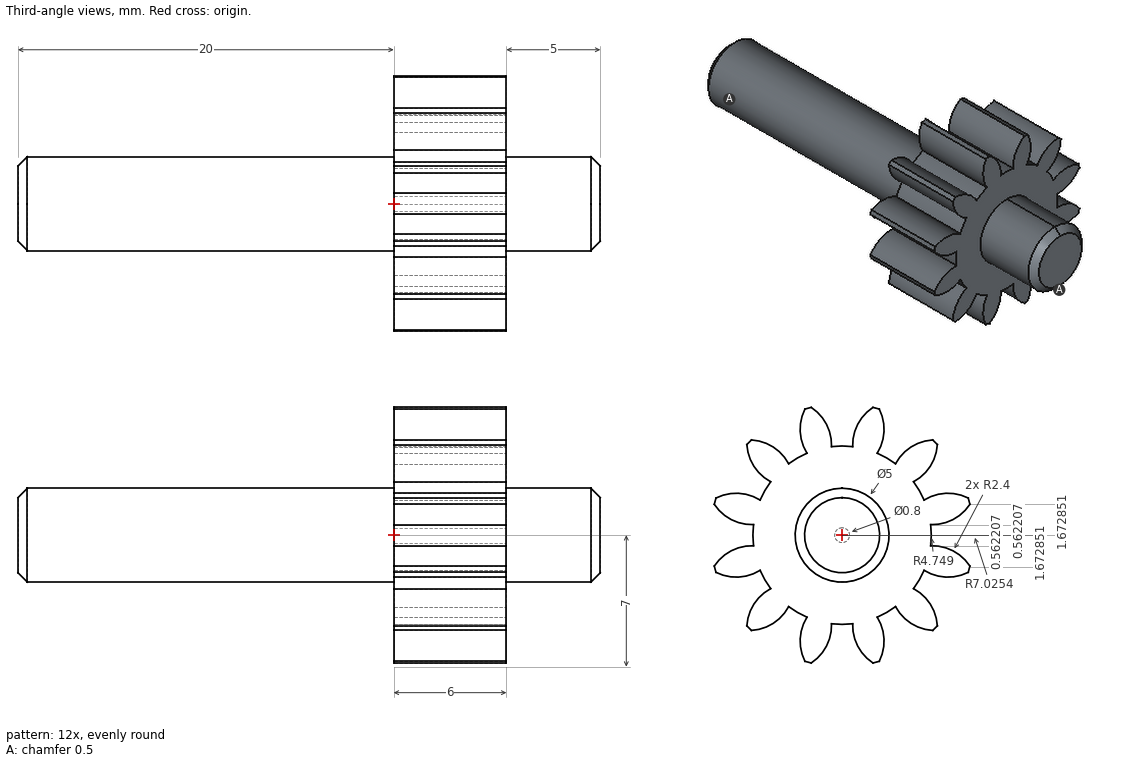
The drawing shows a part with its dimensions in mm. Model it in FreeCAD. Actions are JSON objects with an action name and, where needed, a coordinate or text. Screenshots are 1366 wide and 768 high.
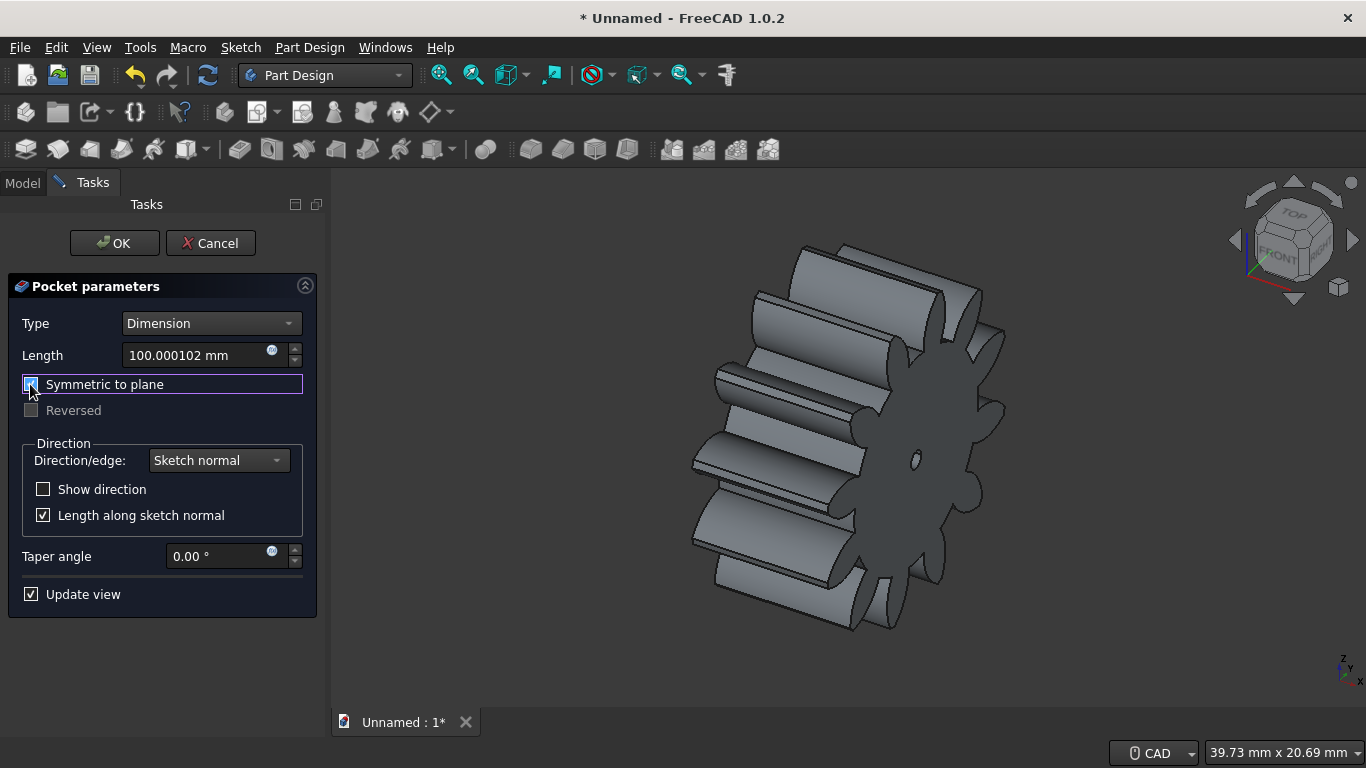
{"action": "left_click", "coordinate": [115, 243]}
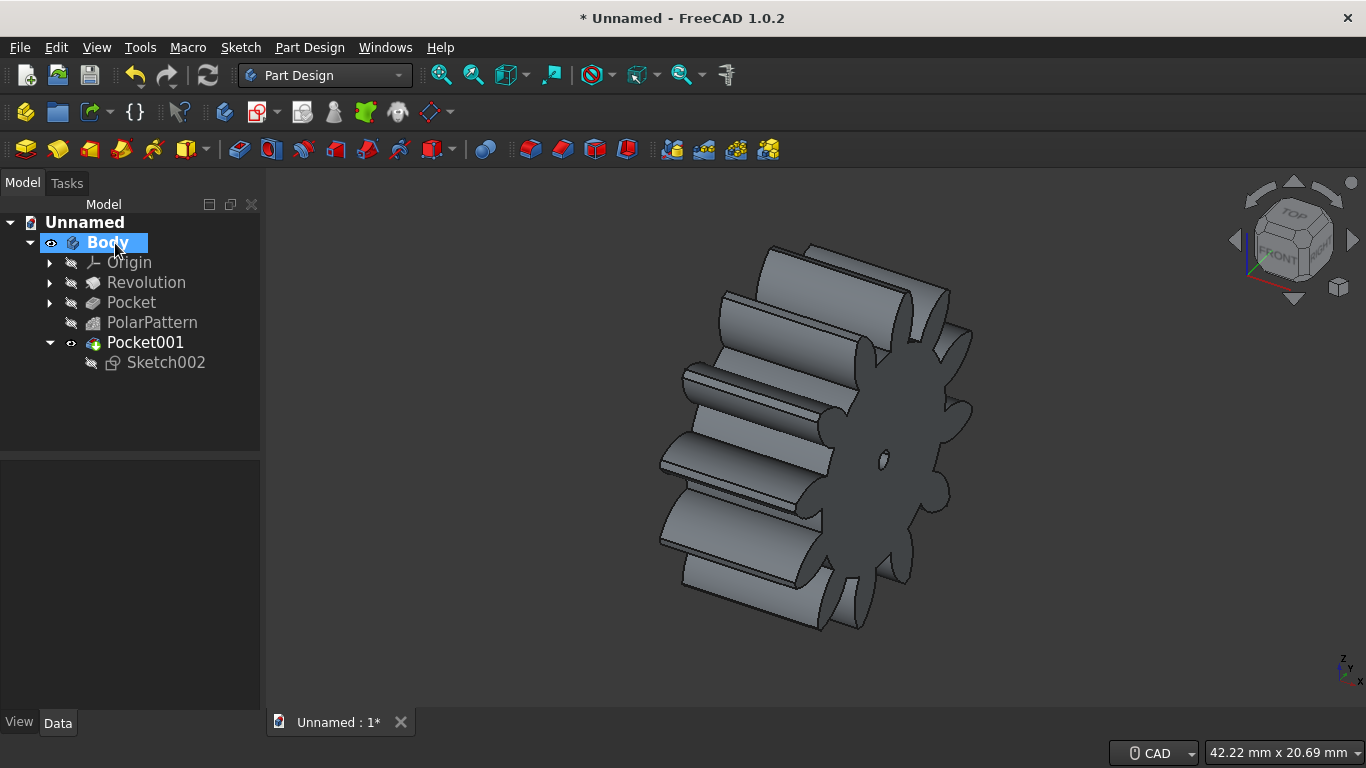
{"action": "left_click", "coordinate": [858, 443]}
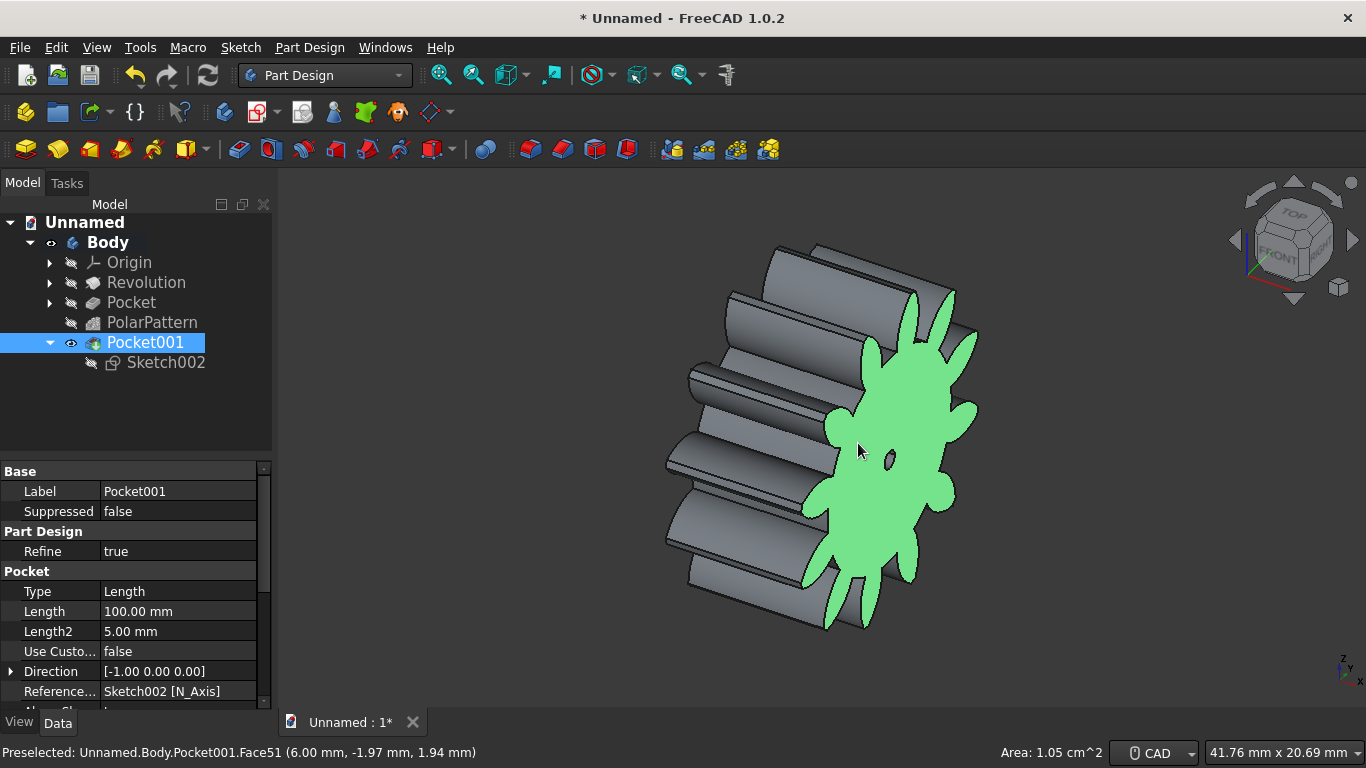
{"action": "left_click", "coordinate": [258, 112]}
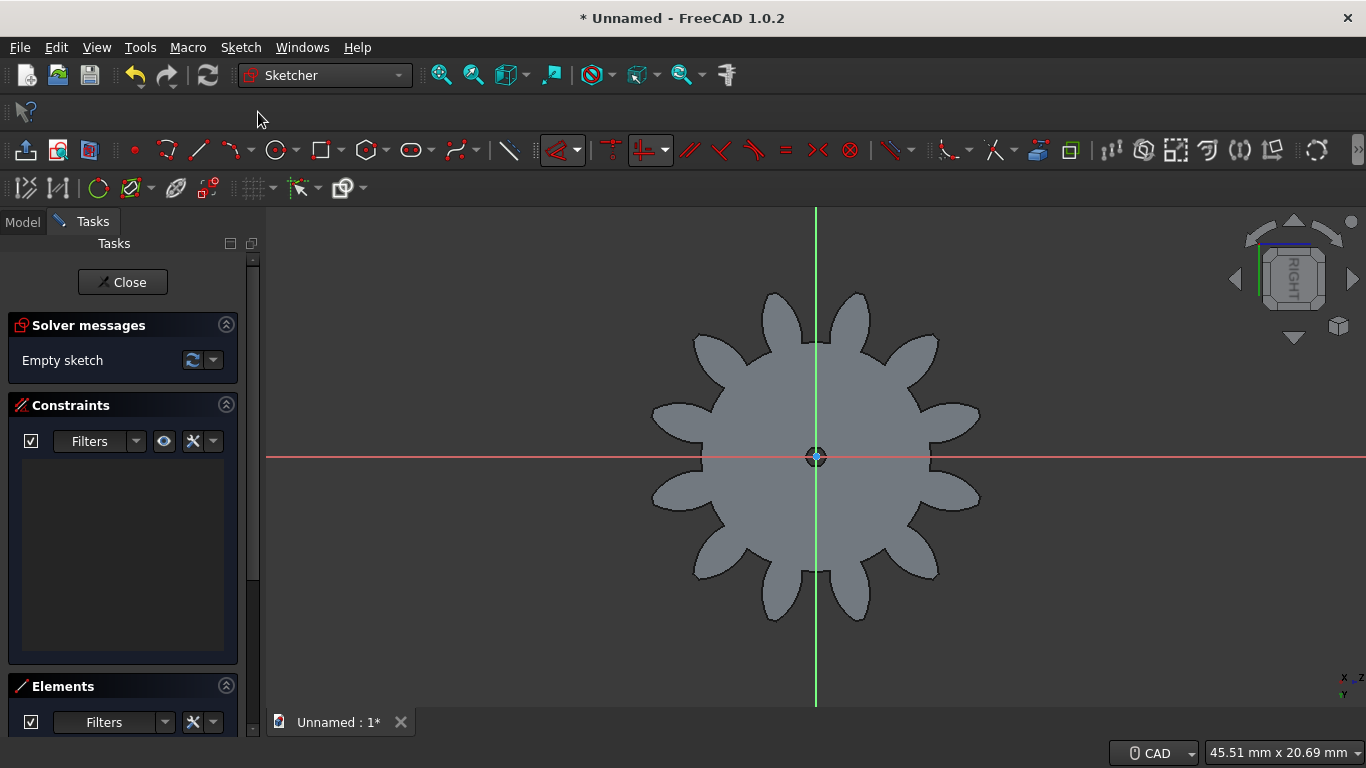
{"action": "scroll", "coordinate": [856, 457], "scroll_direction": "up", "scroll_amount": 5}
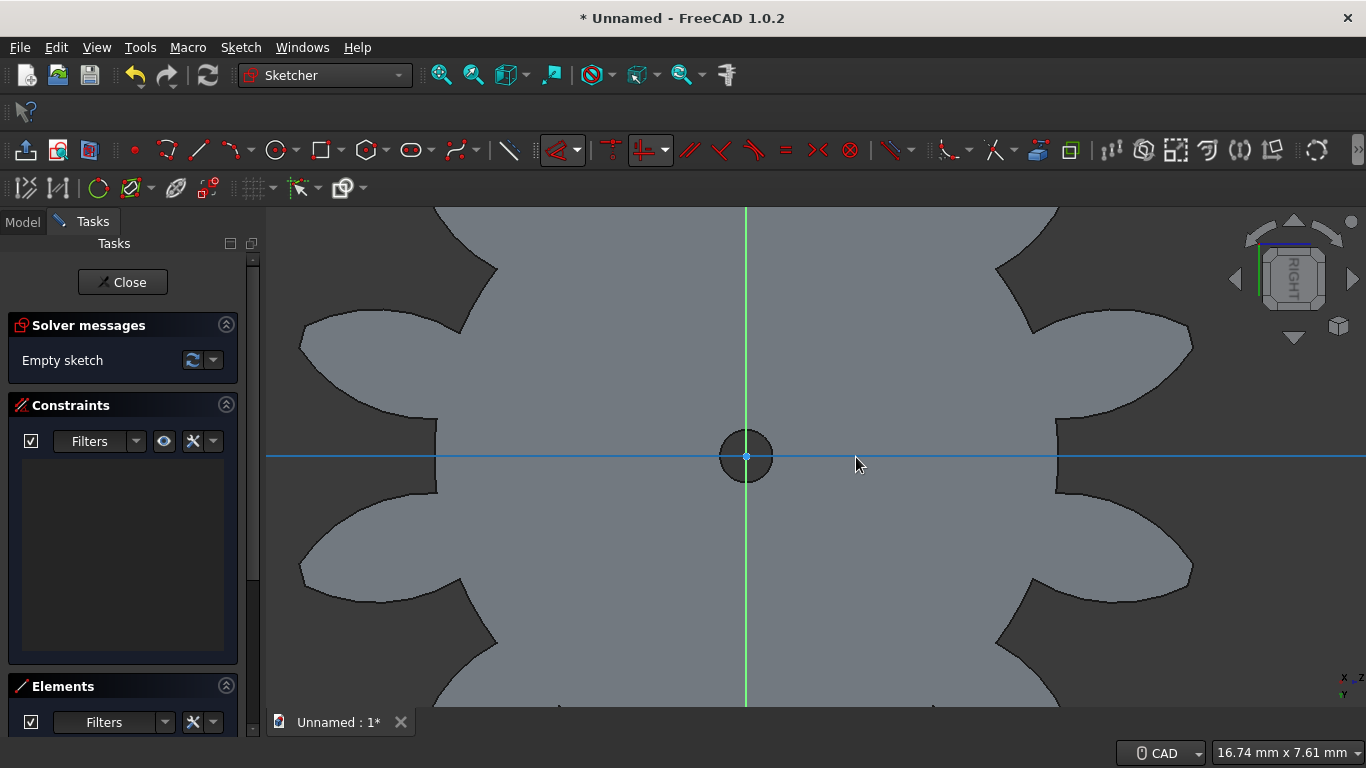
{"action": "left_click", "coordinate": [276, 150]}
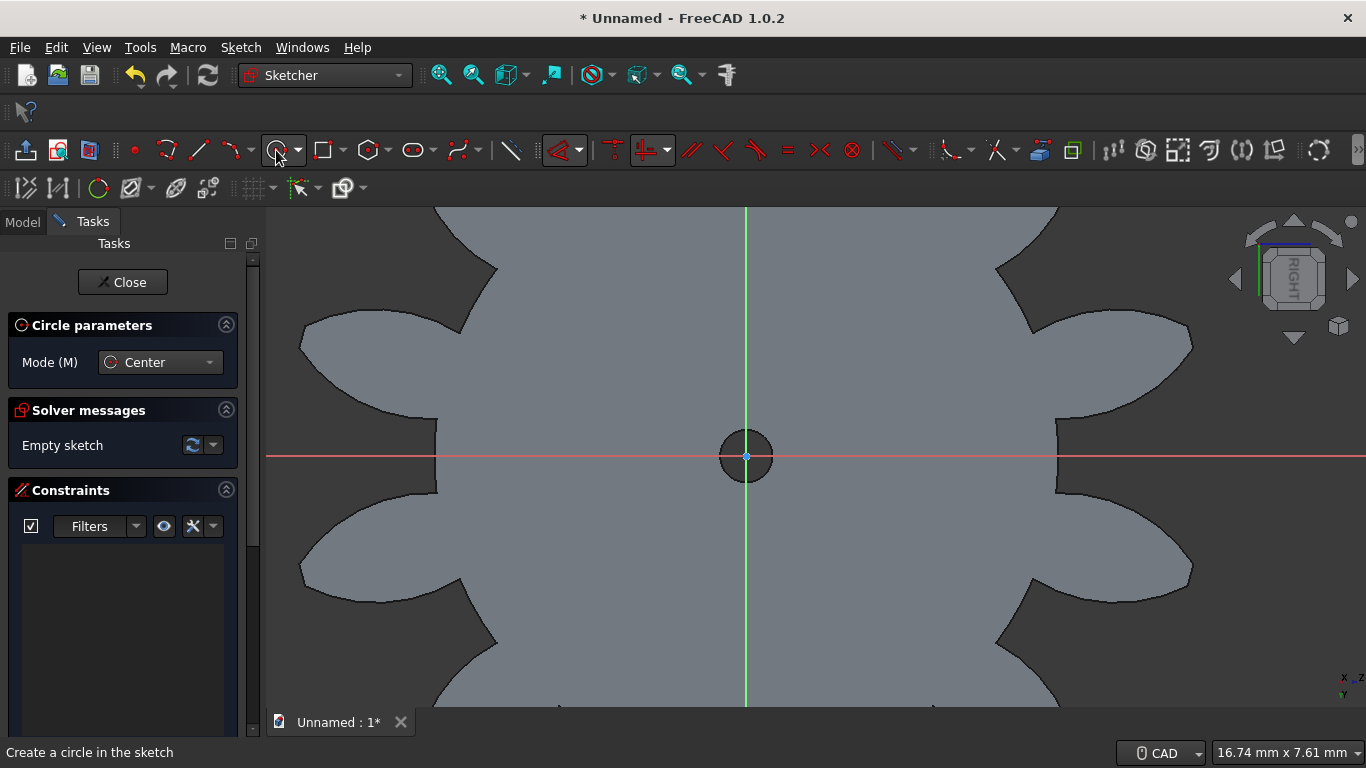
{"action": "left_click", "coordinate": [746, 456]}
{"action": "left_click", "coordinate": [862, 340]}
{"action": "key", "text": "Escape"}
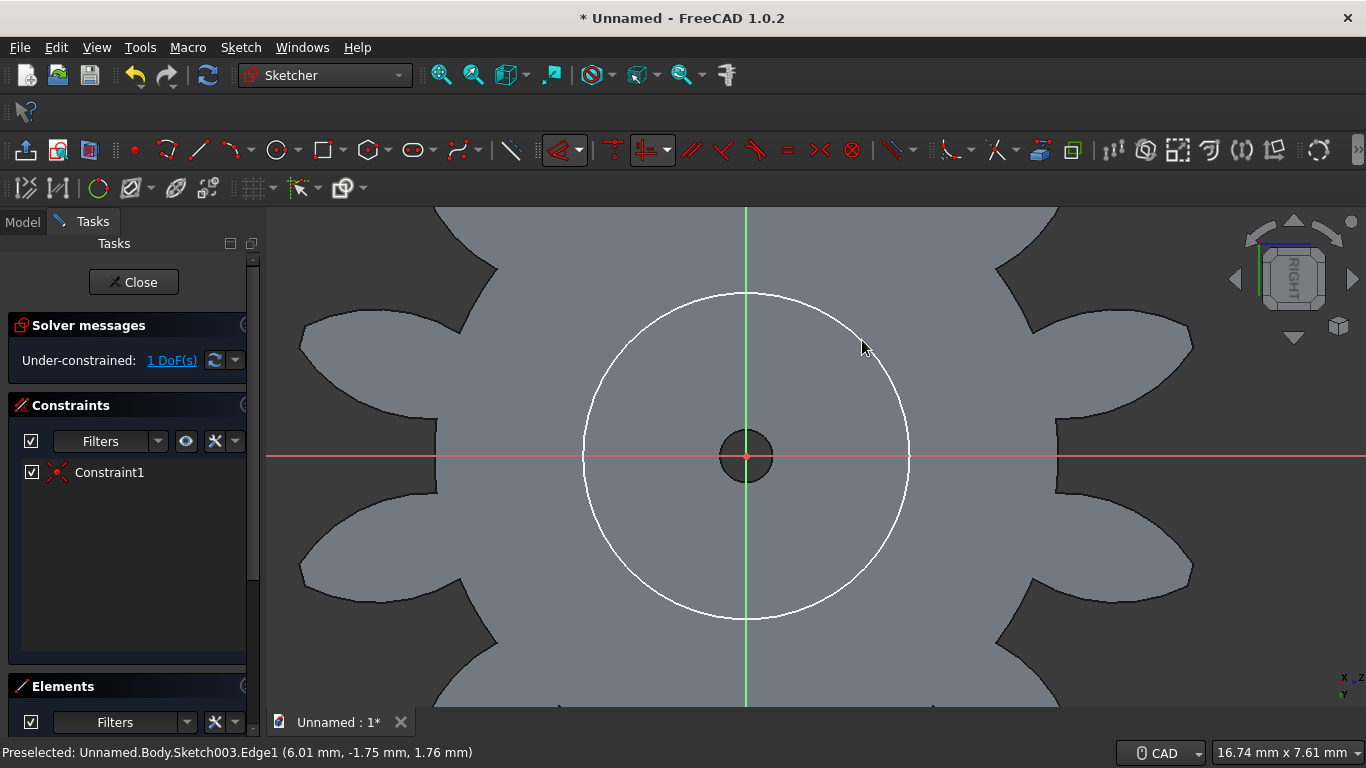
{"action": "left_click", "coordinate": [861, 340]}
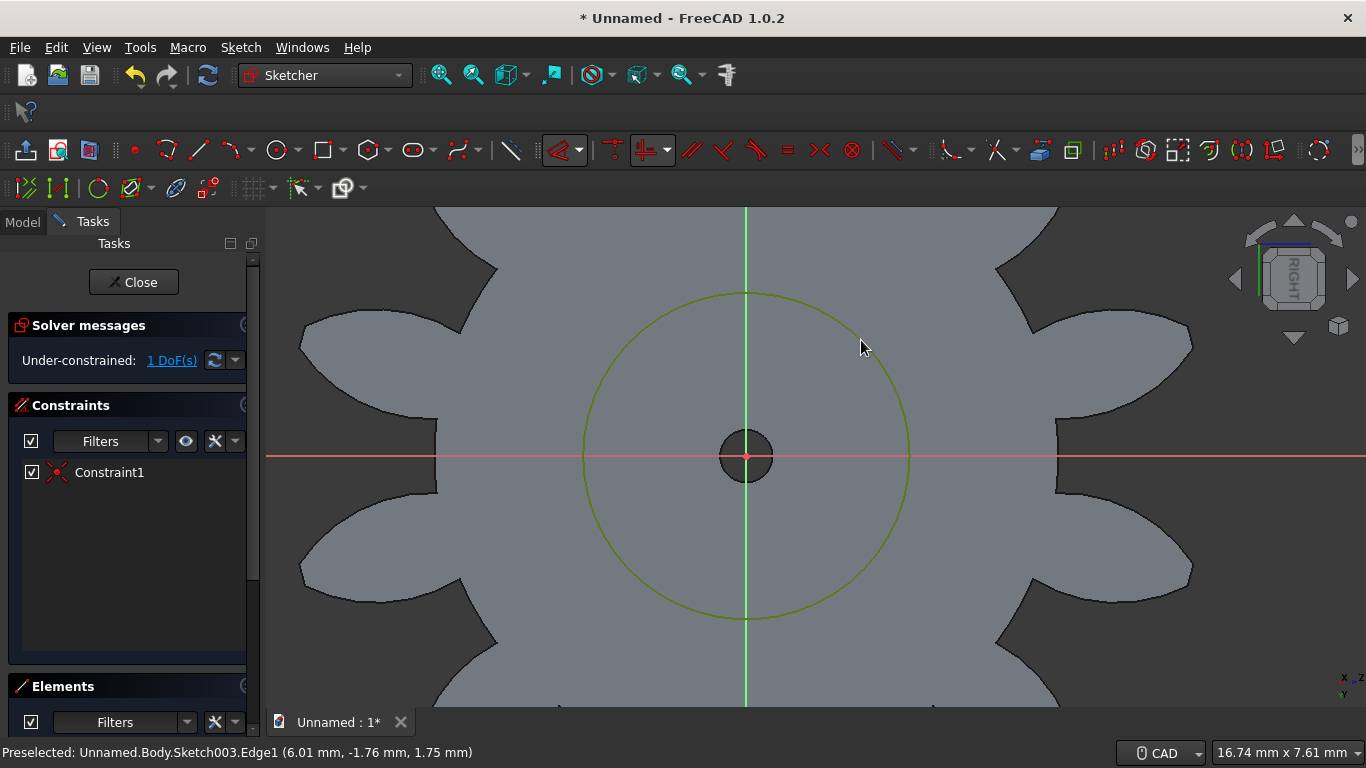
{"action": "left_click", "coordinate": [582, 150]}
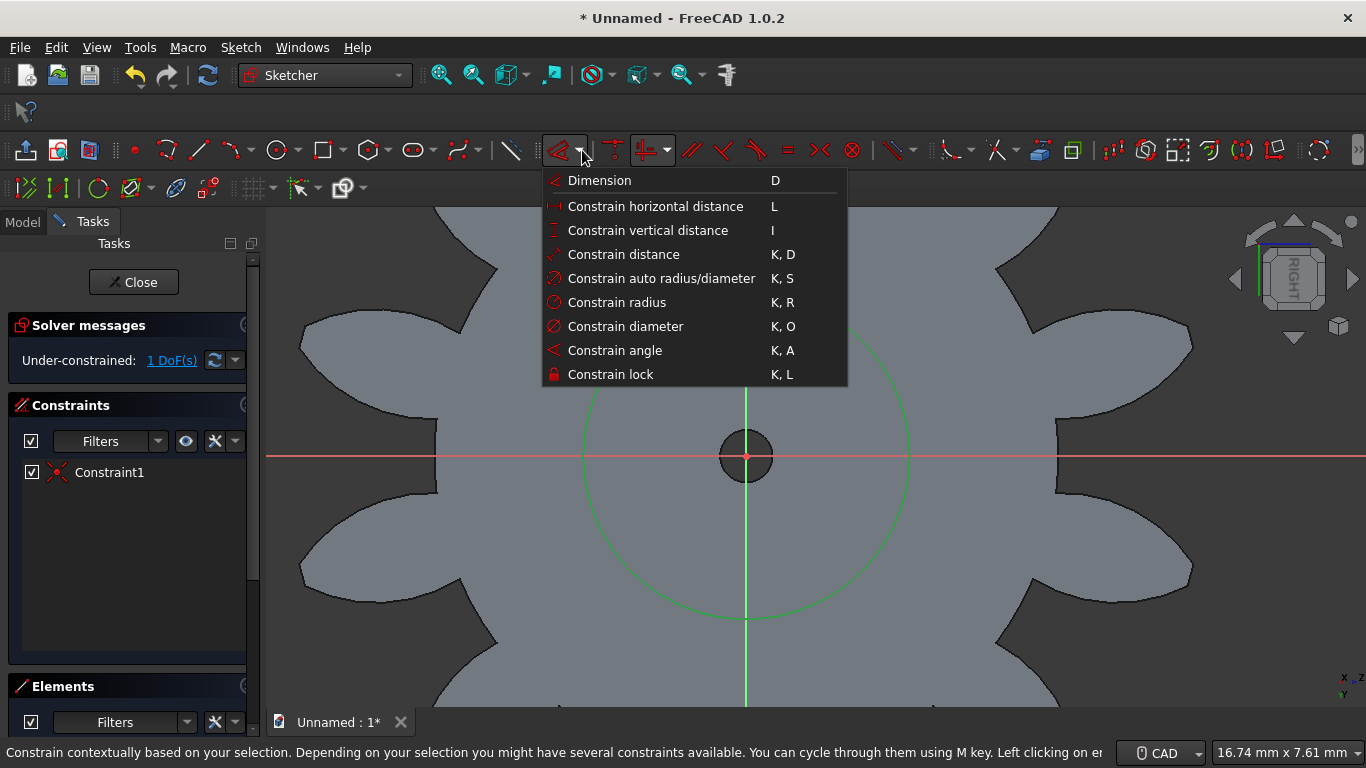
{"action": "left_click", "coordinate": [695, 326]}